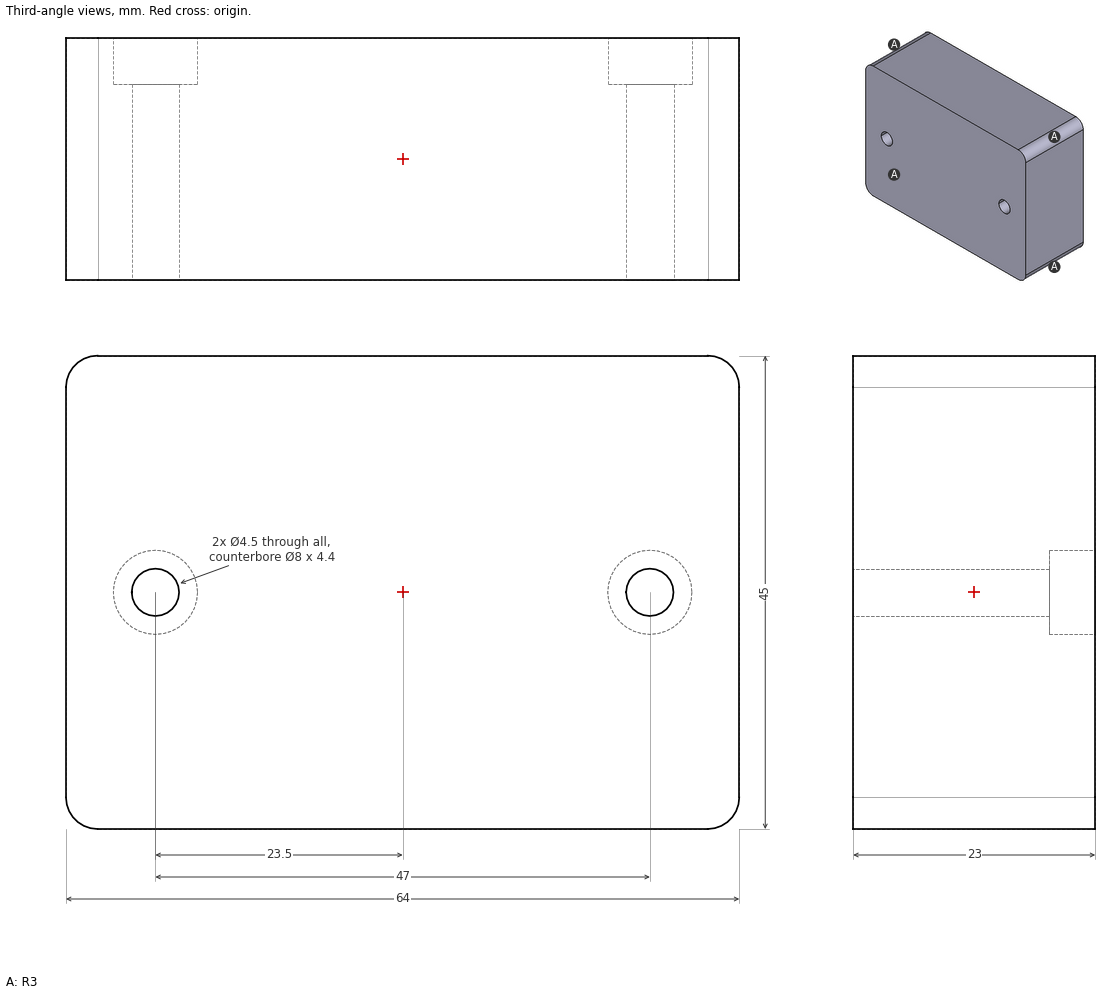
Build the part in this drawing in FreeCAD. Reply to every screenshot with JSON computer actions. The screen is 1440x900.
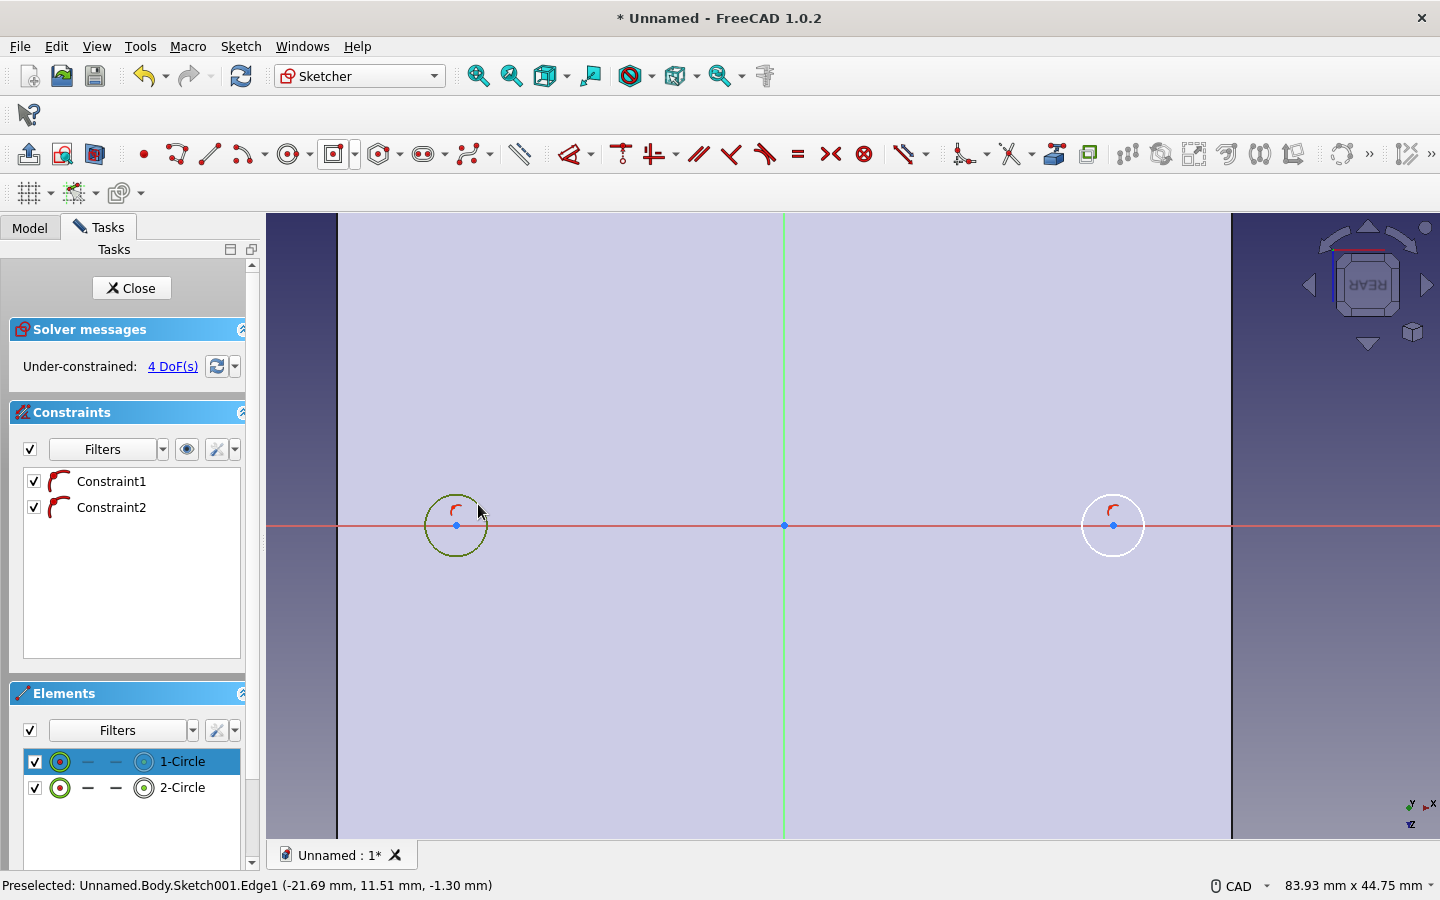
{"action": "left_click", "coordinate": [1135, 504]}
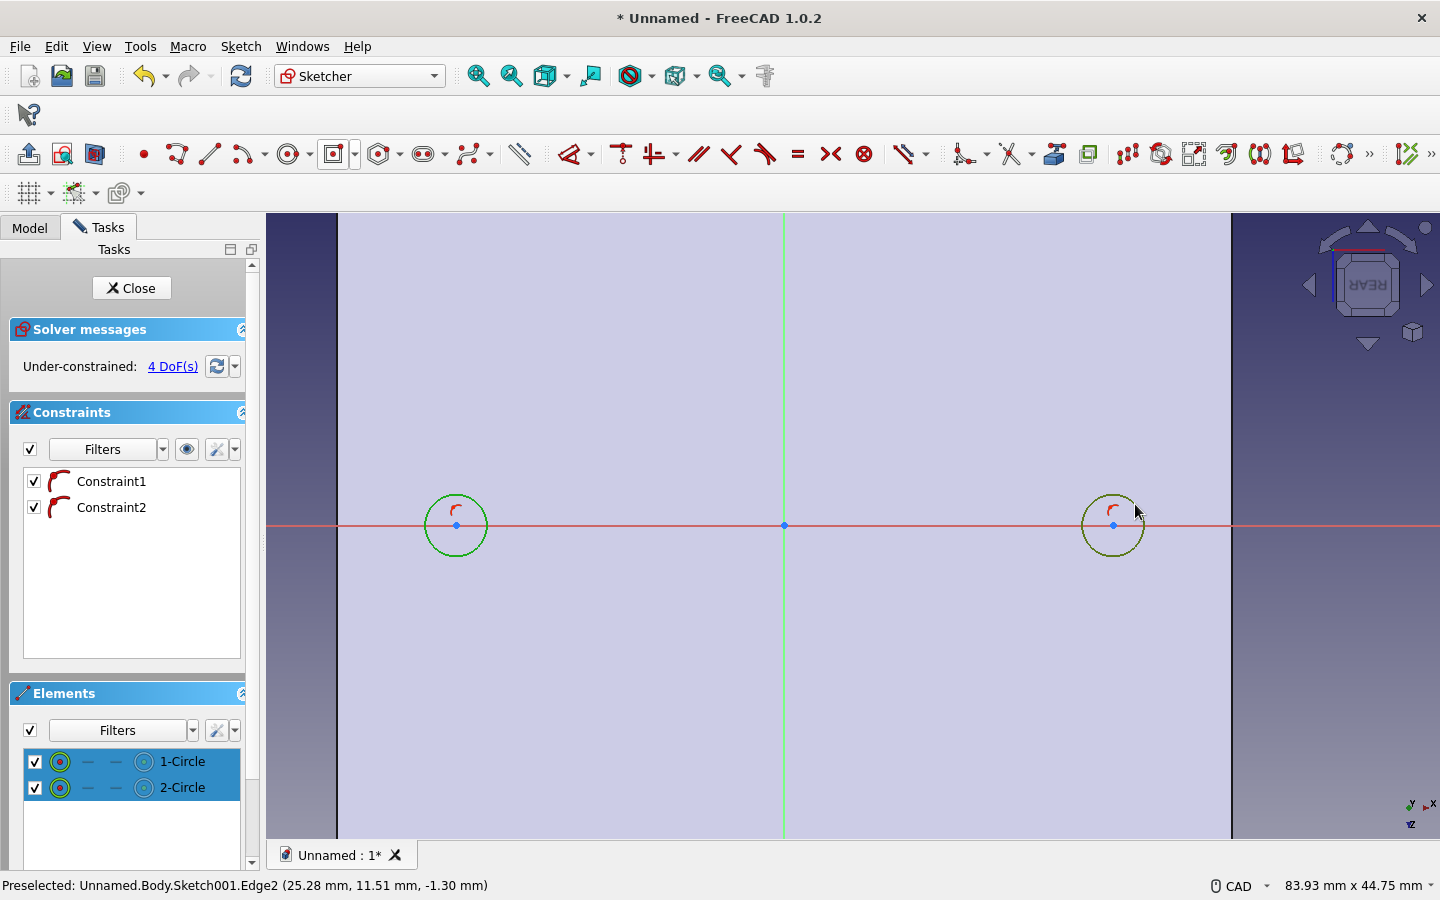
{"action": "key", "text": "e"}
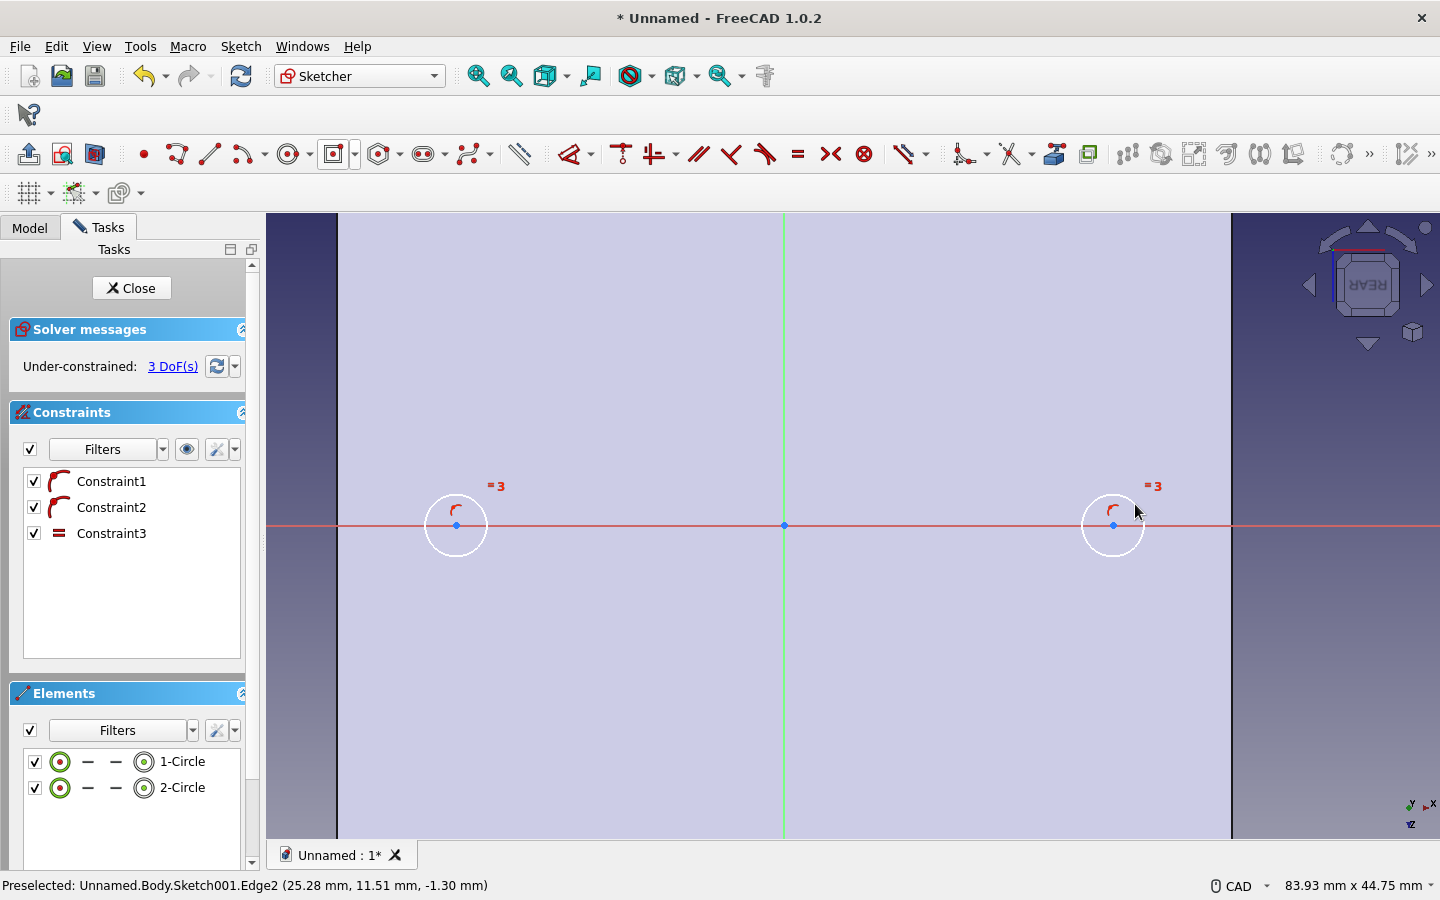
{"action": "left_click", "coordinate": [478, 504]}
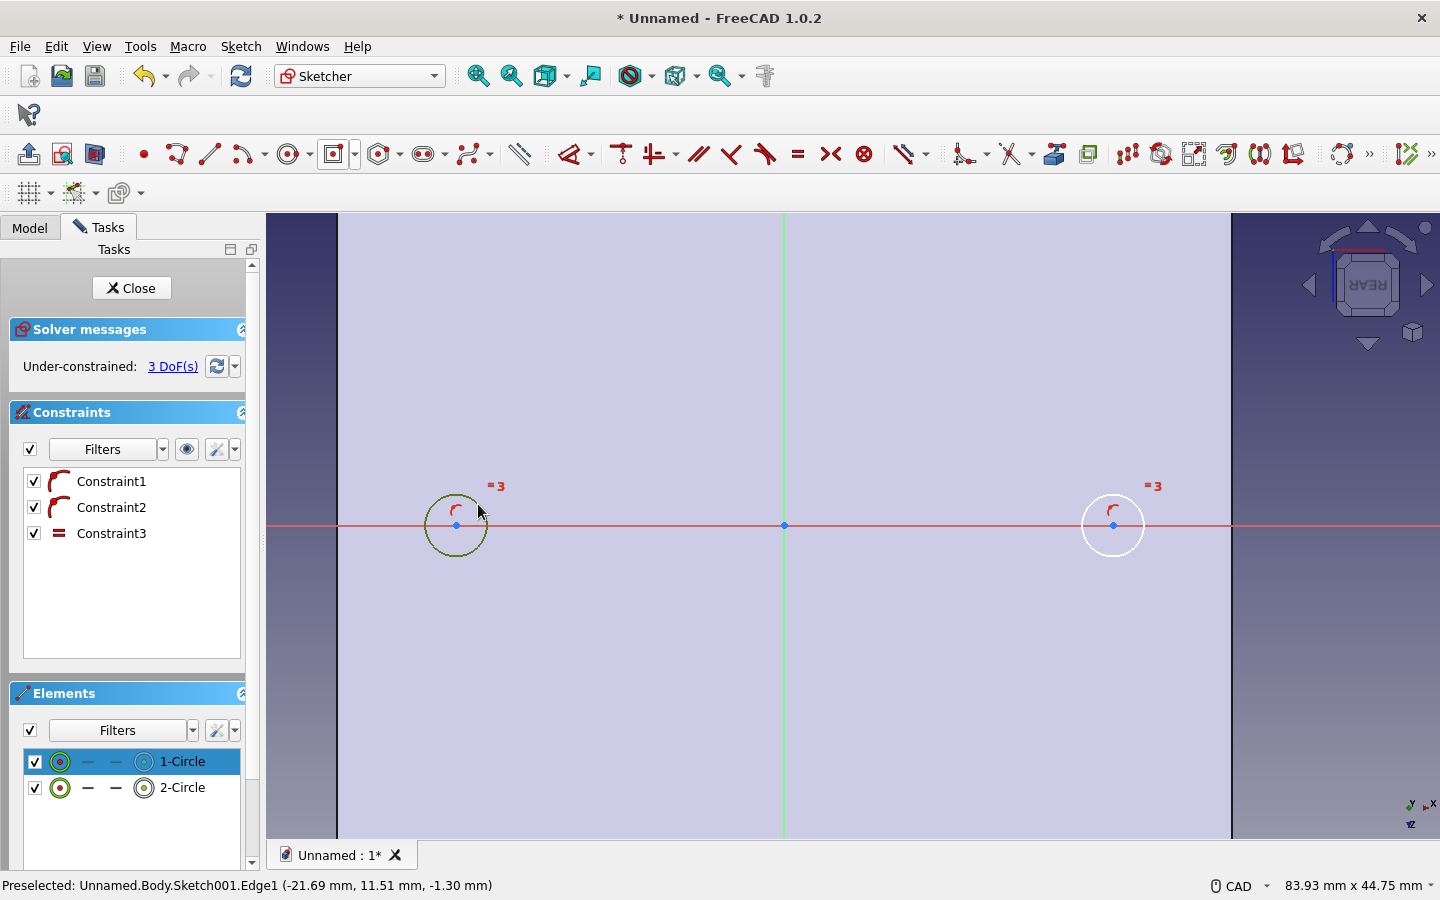
{"action": "key", "text": "k o"}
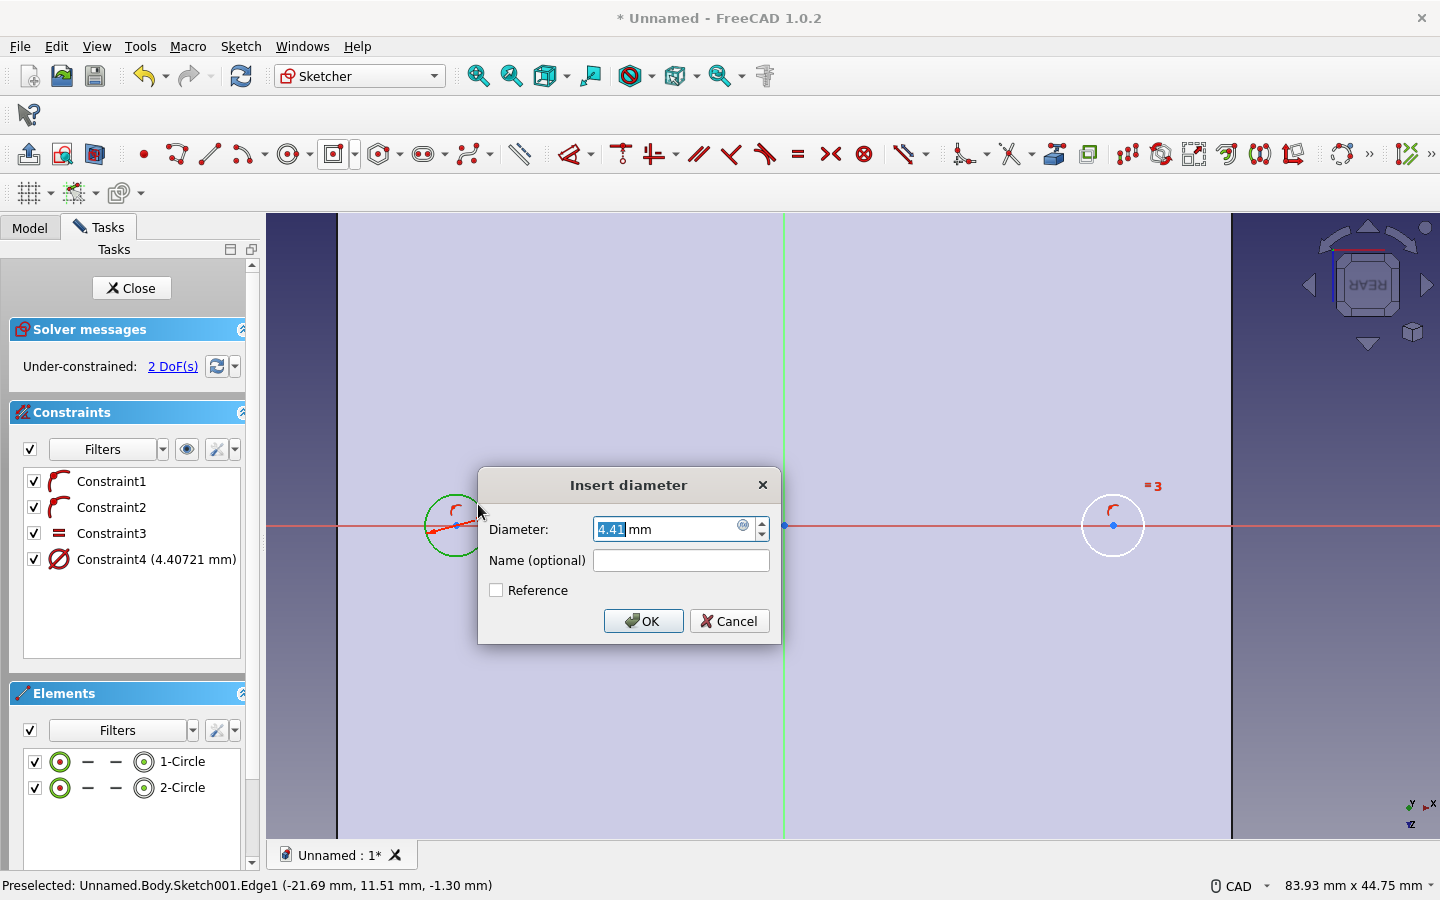
{"action": "type", "text": "4.5"}
{"action": "key", "text": "Return"}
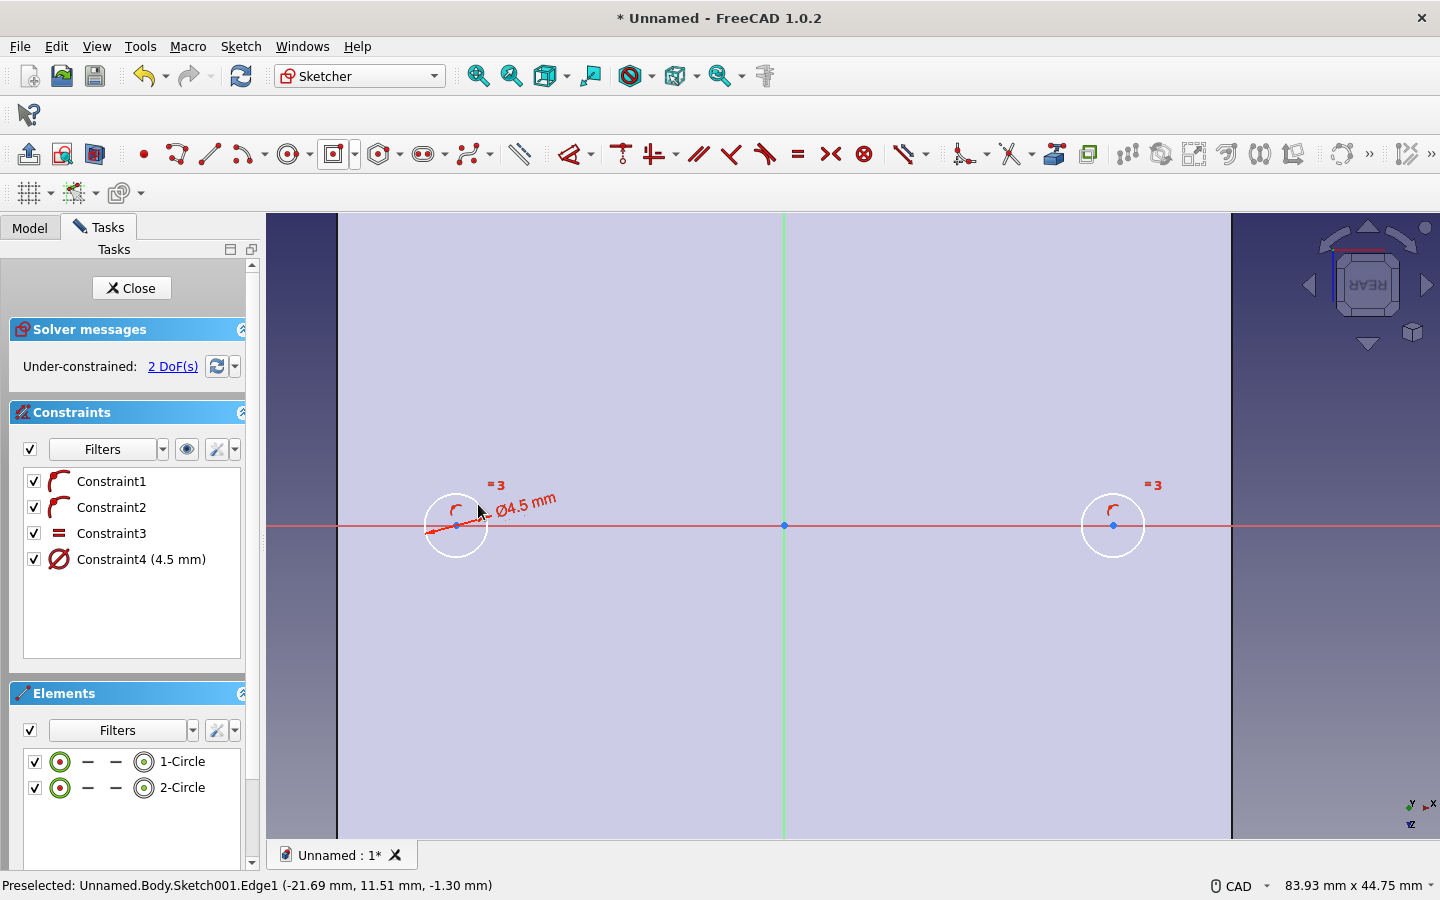
{"action": "left_click", "coordinate": [456, 526]}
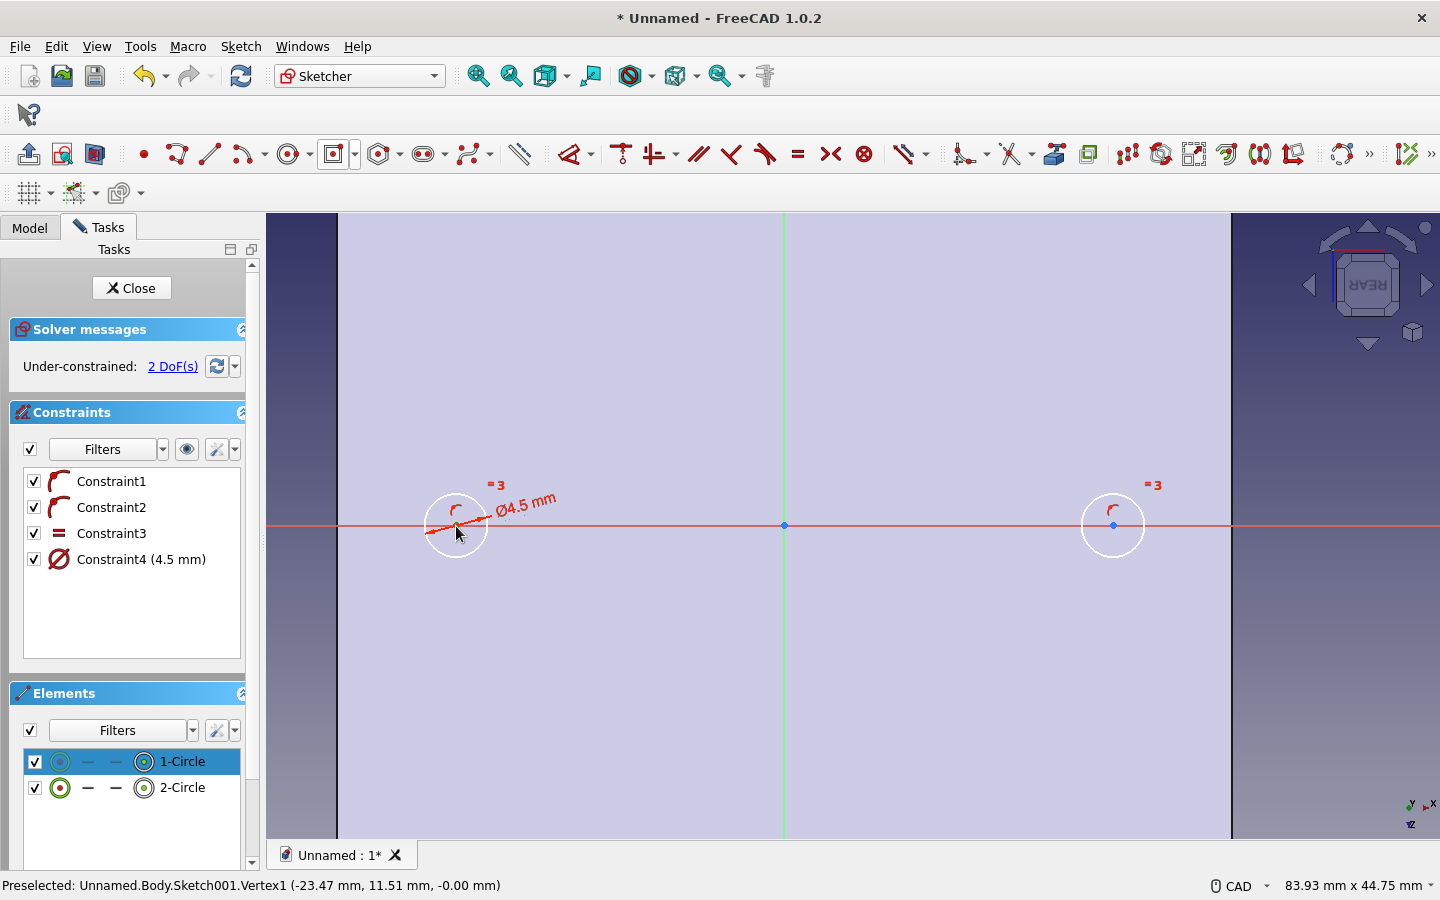
{"action": "left_click", "coordinate": [1113, 526]}